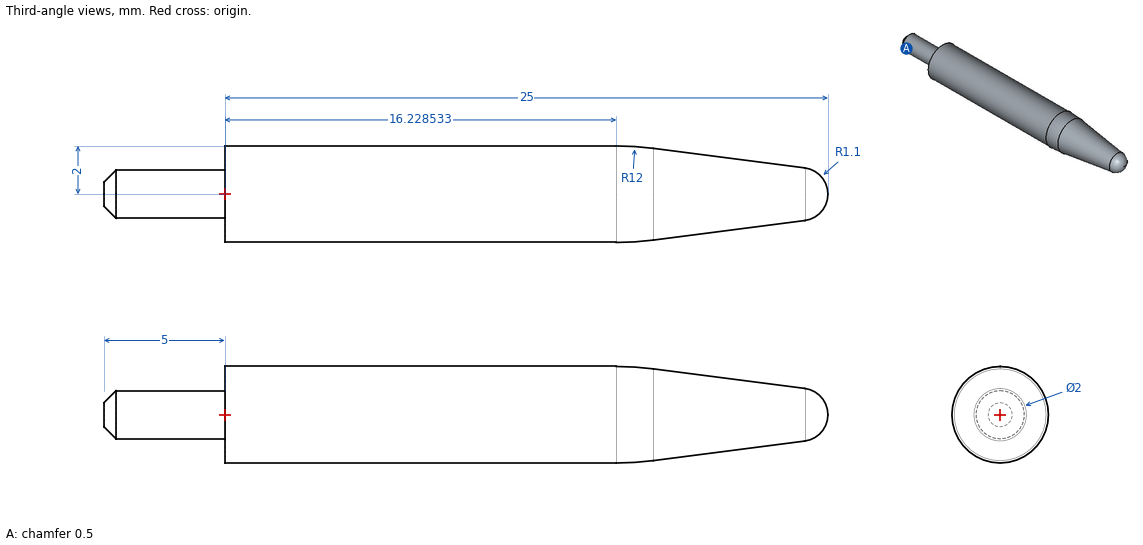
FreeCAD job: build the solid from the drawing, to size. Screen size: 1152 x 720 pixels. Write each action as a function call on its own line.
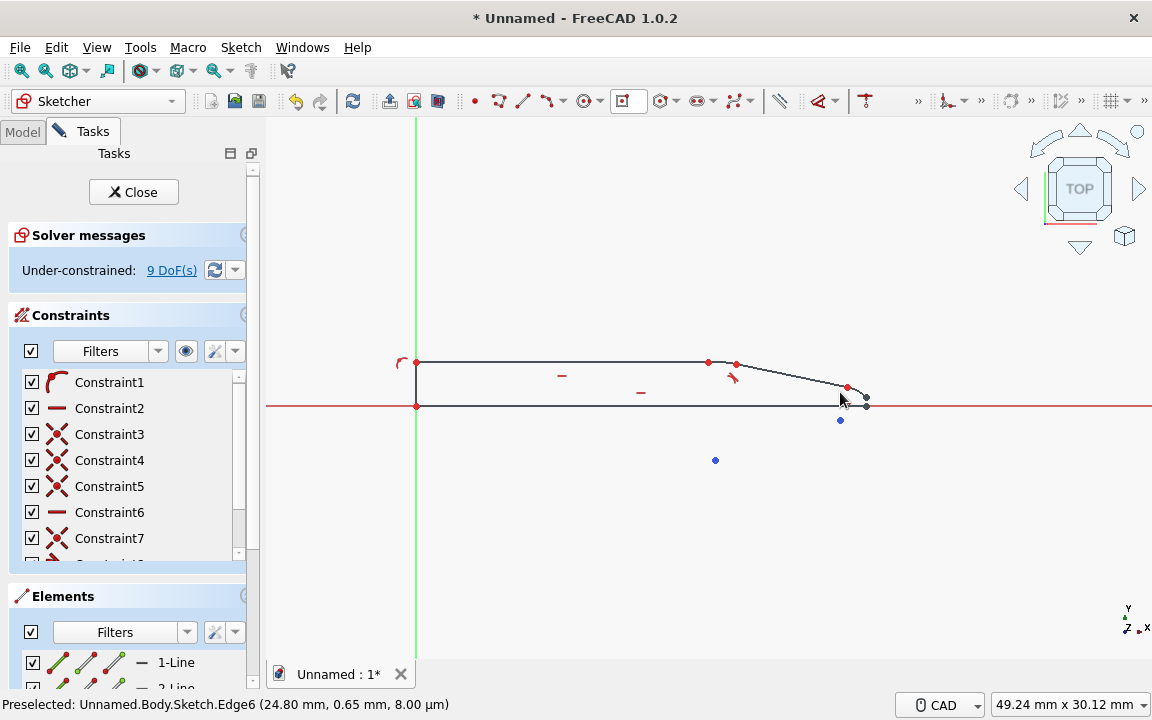
click(621, 362)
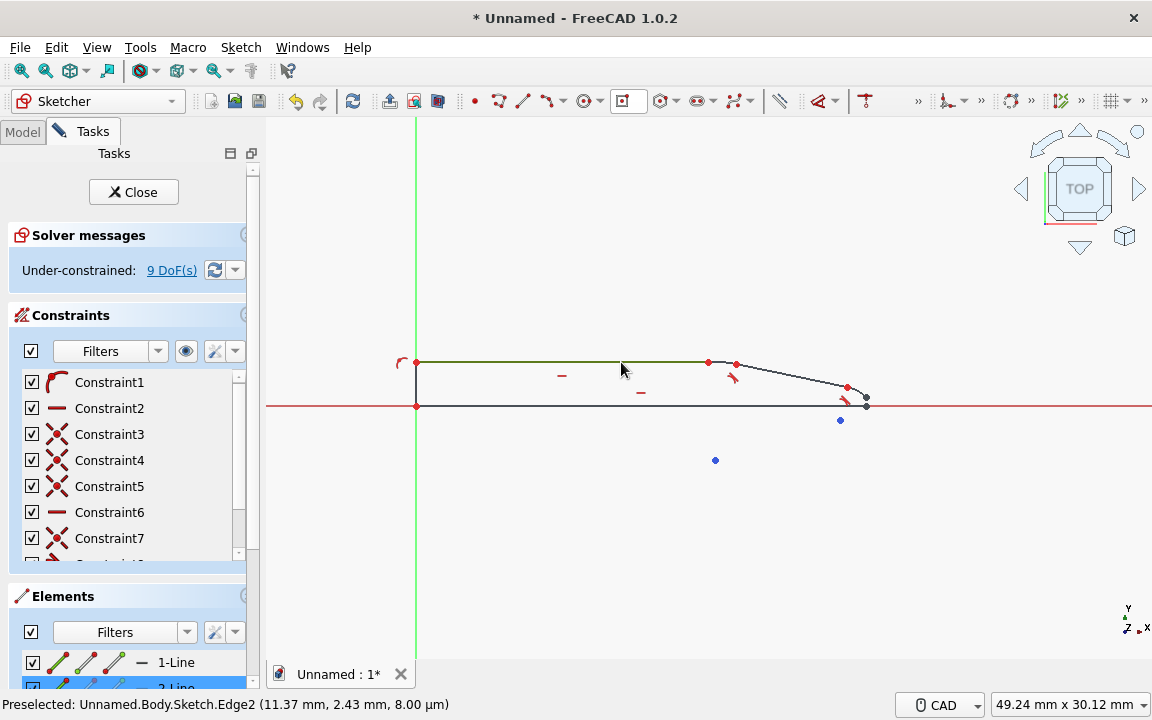
click(722, 362)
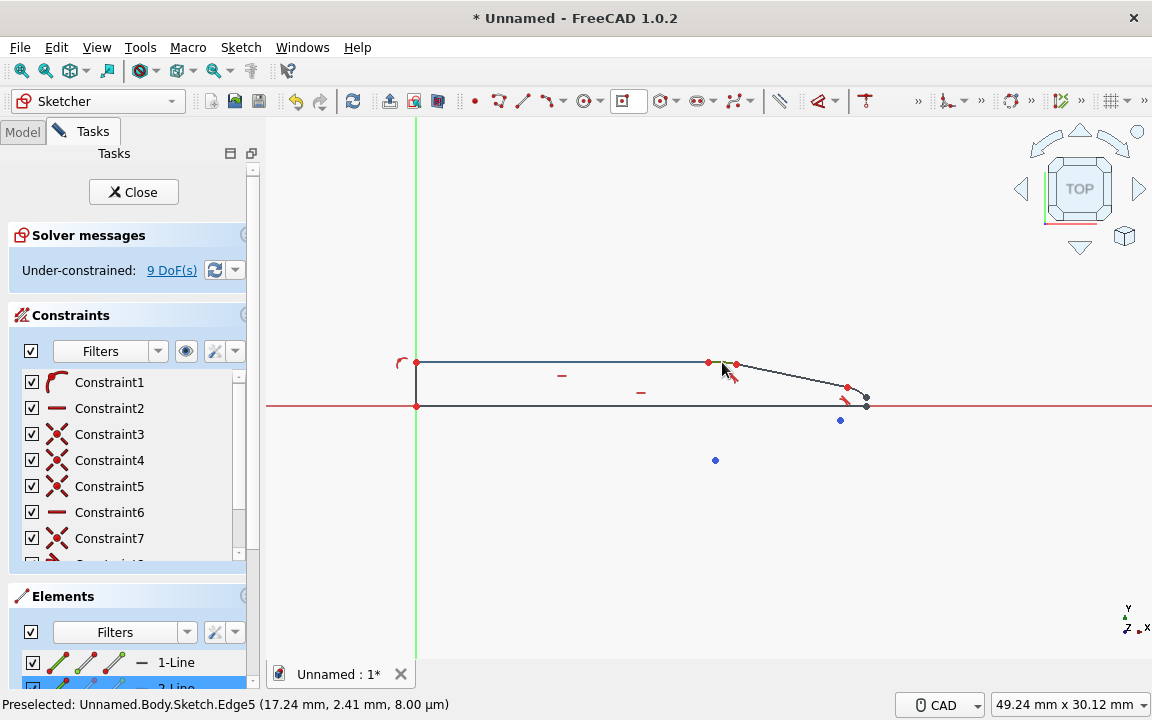
key(t)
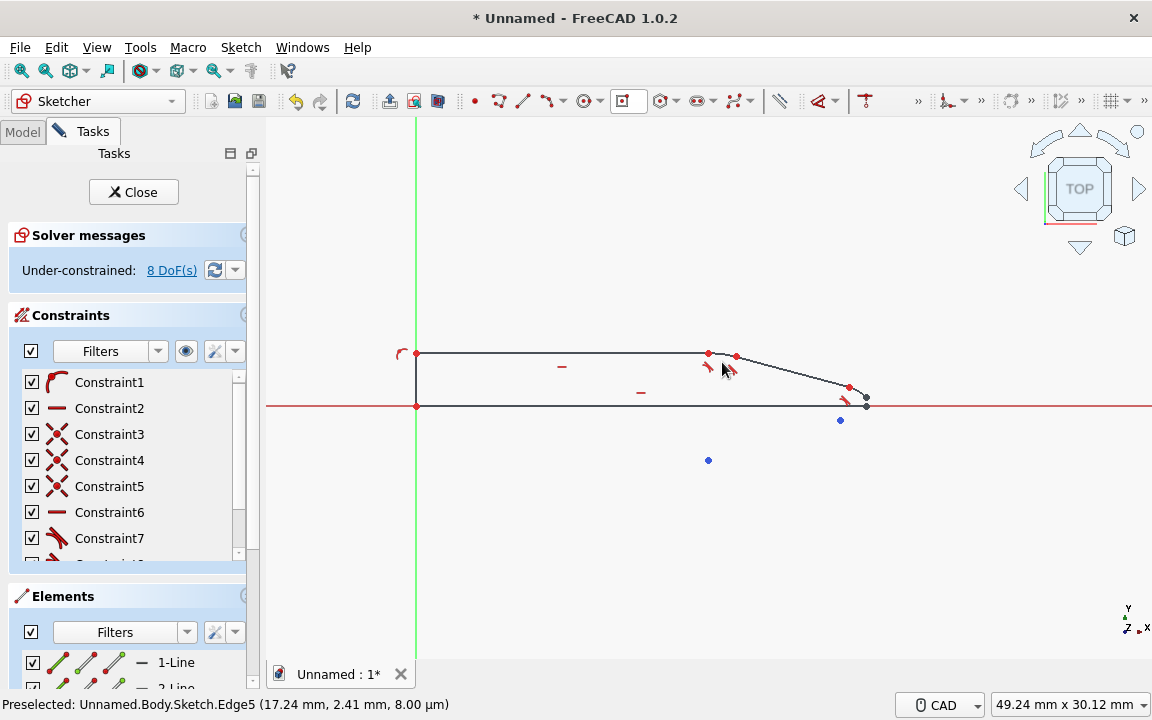
click(840, 421)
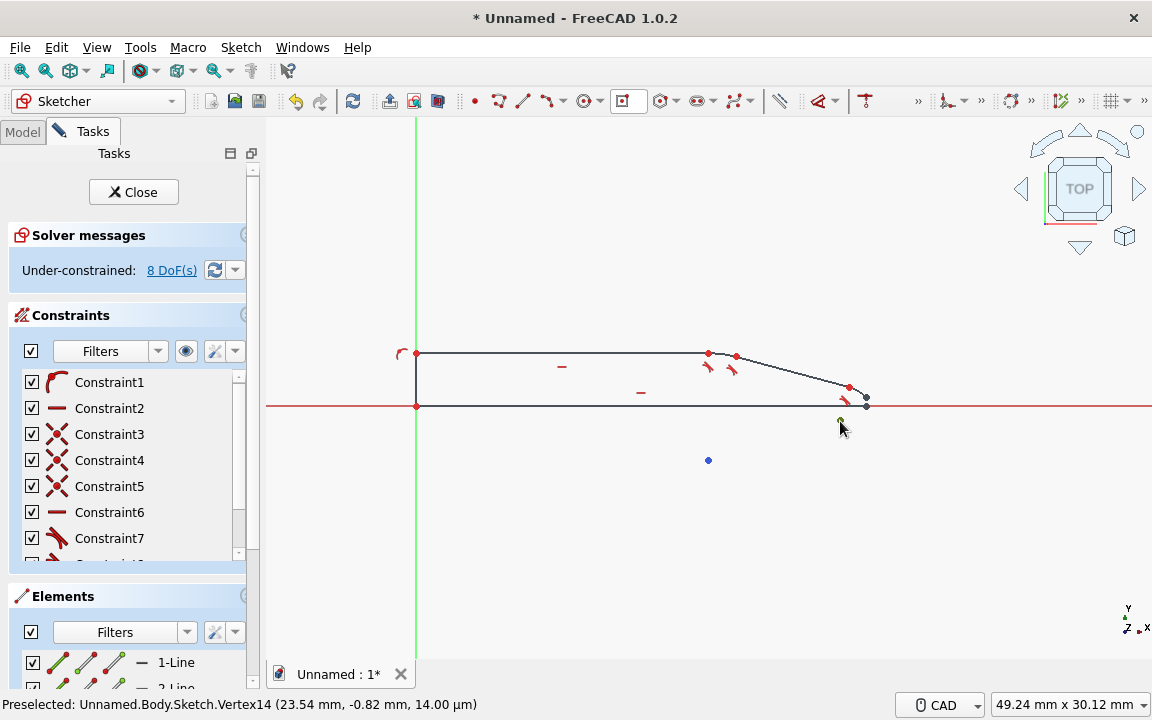
click(344, 406)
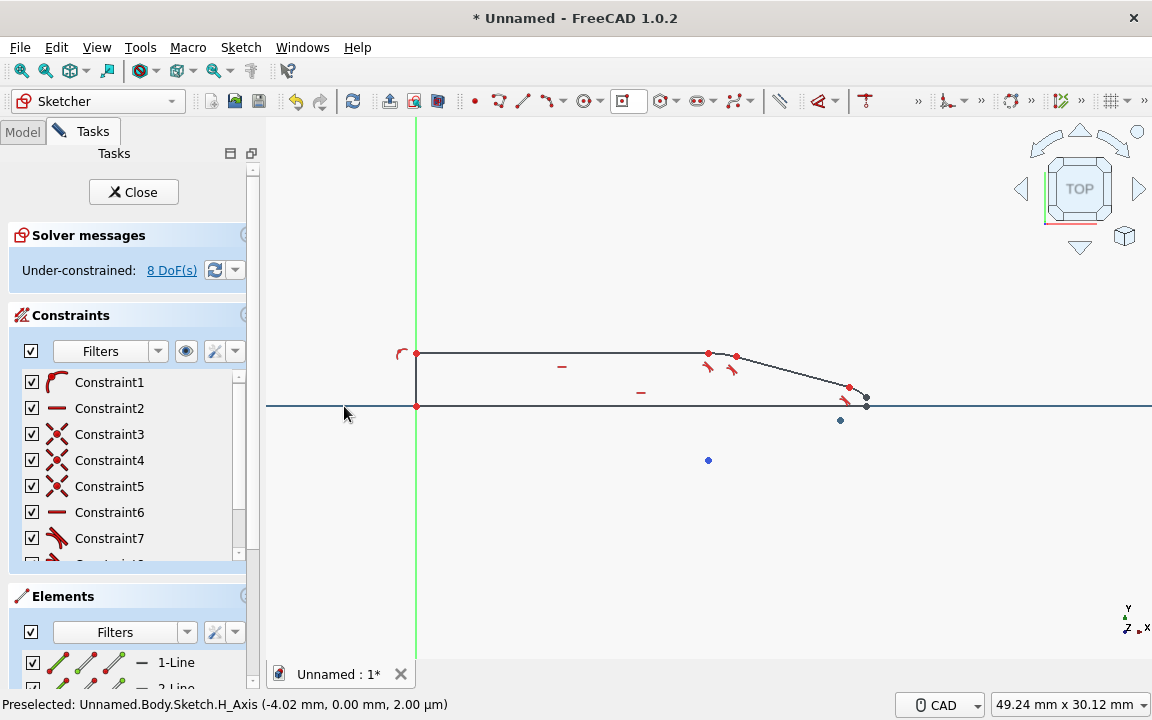
key(c)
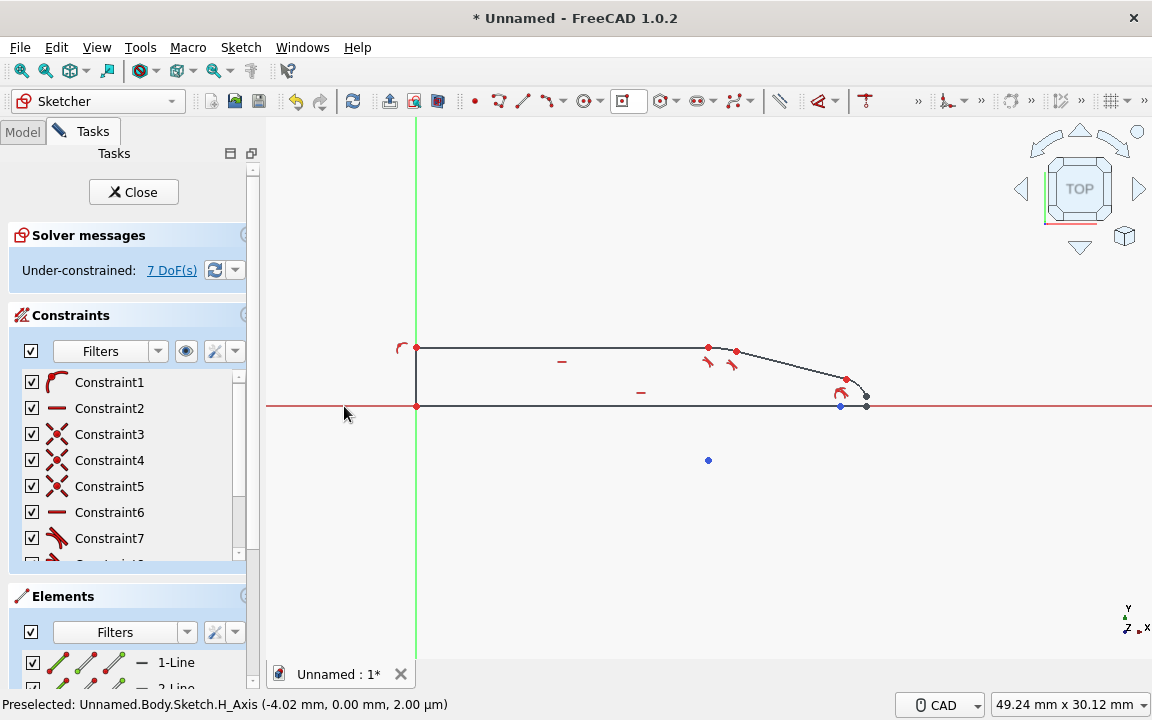
key(d)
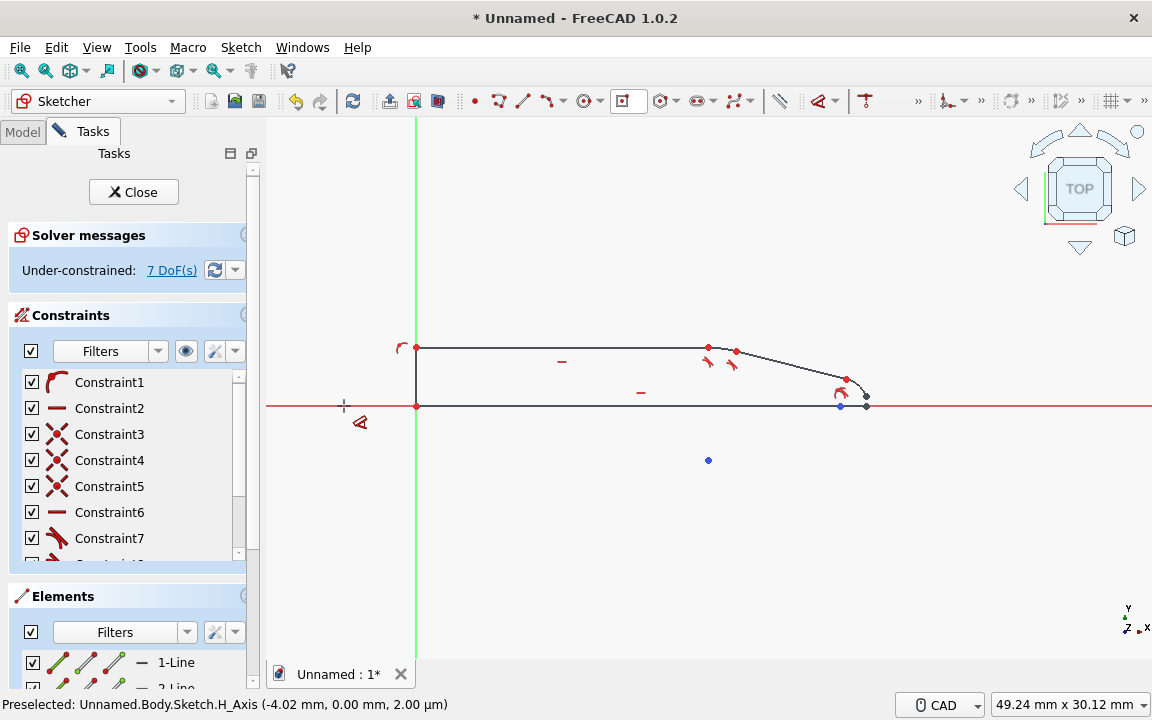
click(722, 349)
click(726, 317)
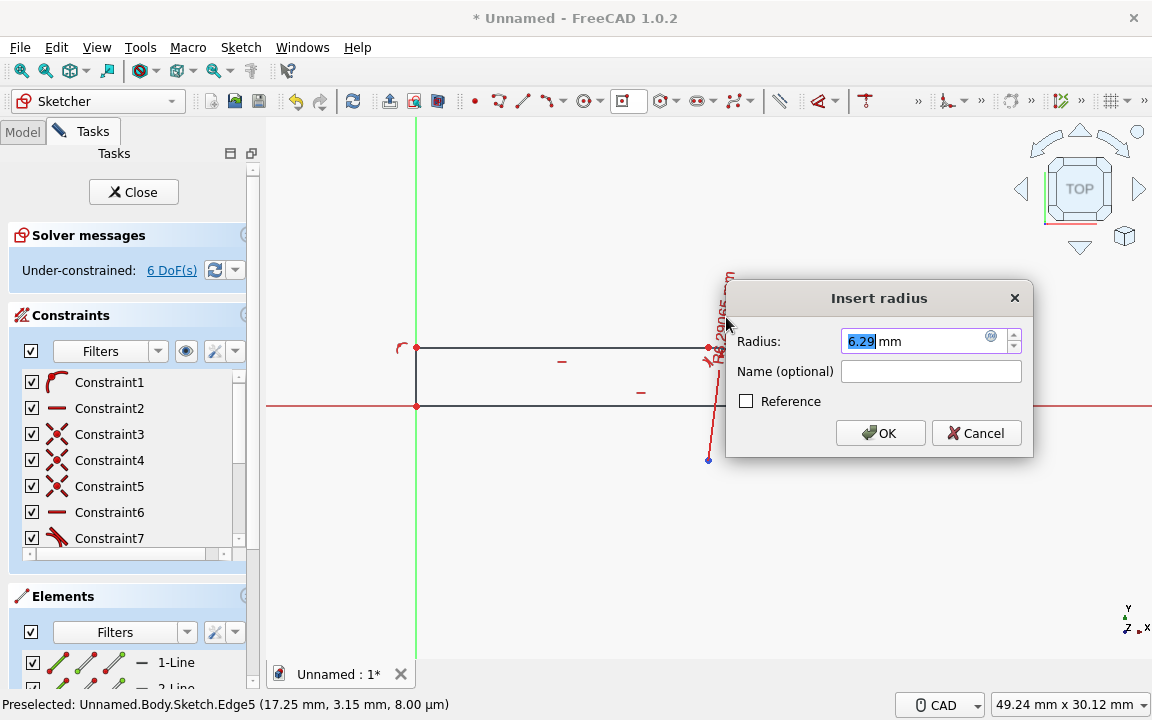
text(12)
key(Return)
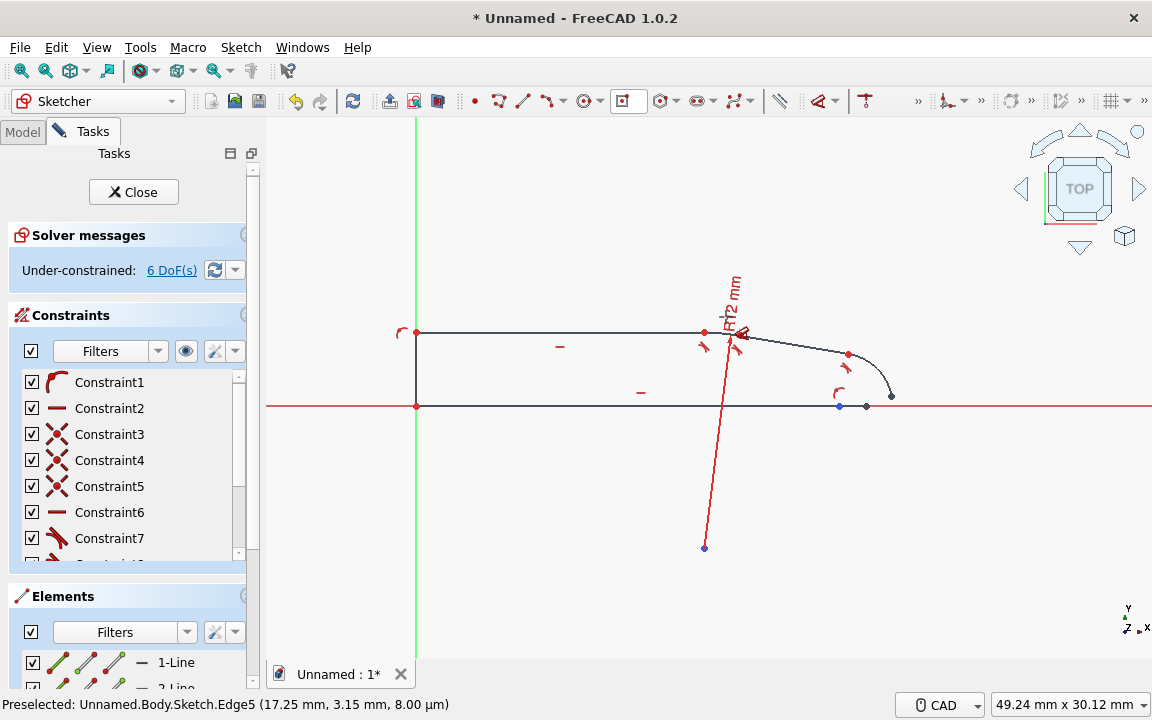
scroll(885, 379, up, 4)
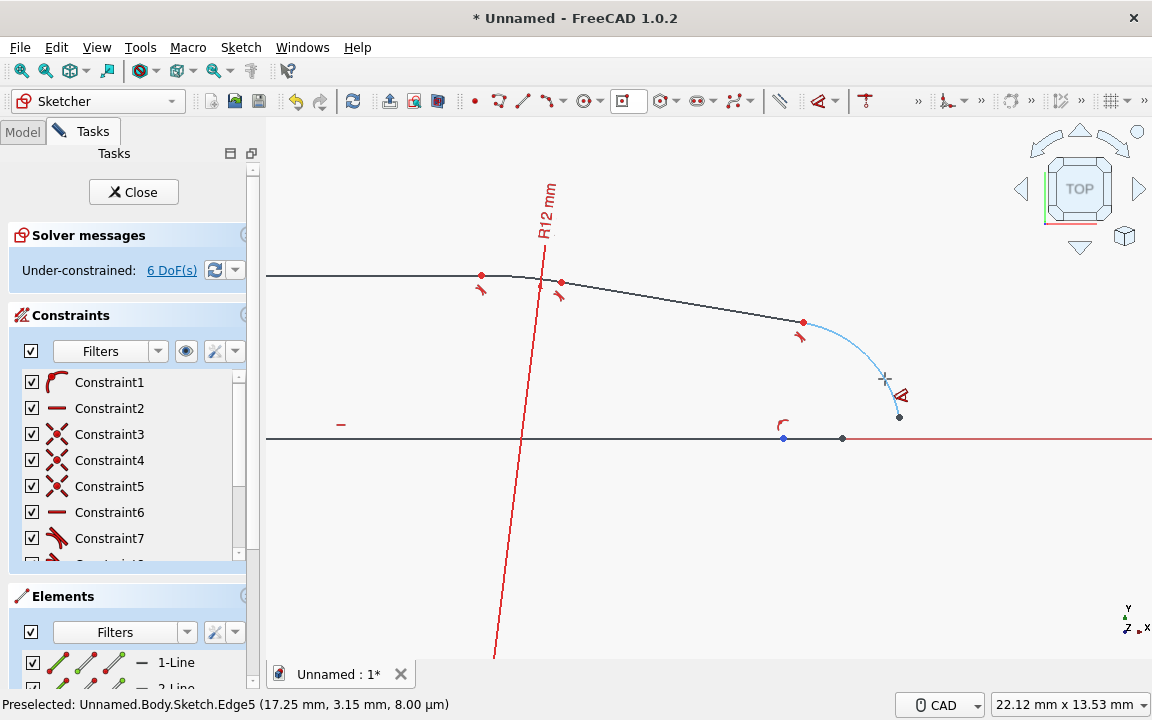
click(884, 378)
click(911, 361)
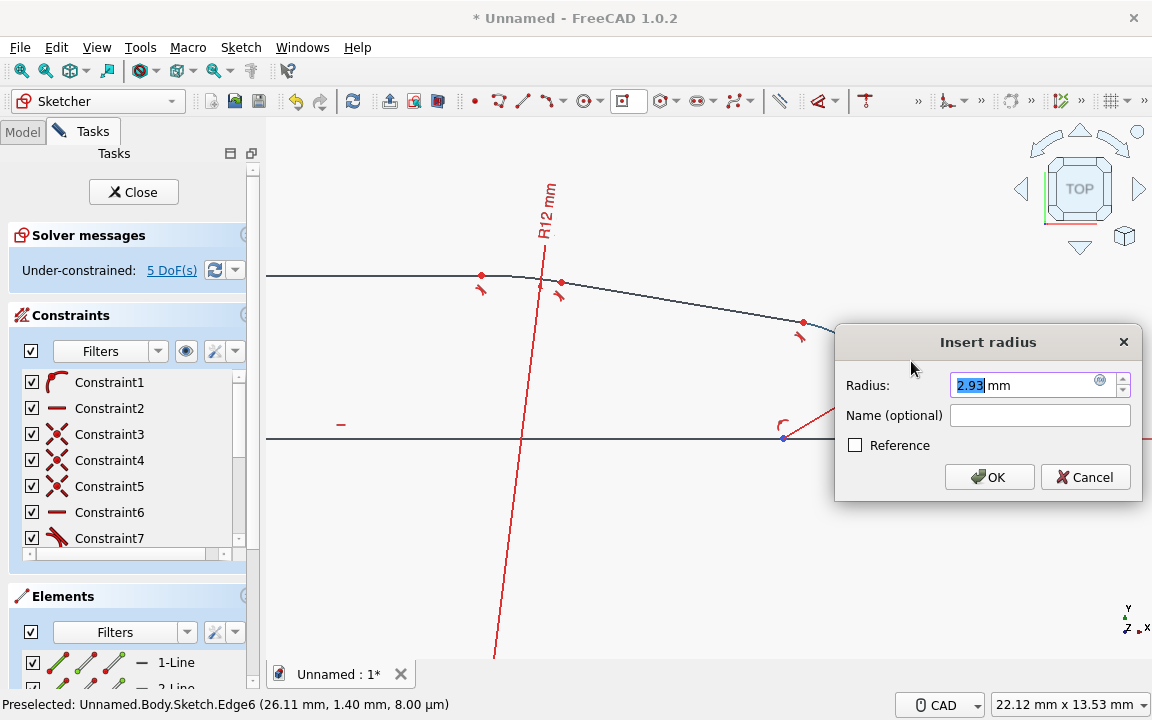
text(1.1)
key(Return)
key(Escape)